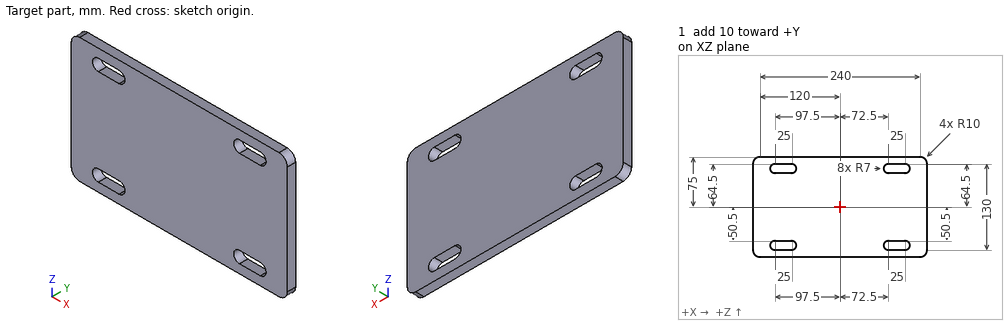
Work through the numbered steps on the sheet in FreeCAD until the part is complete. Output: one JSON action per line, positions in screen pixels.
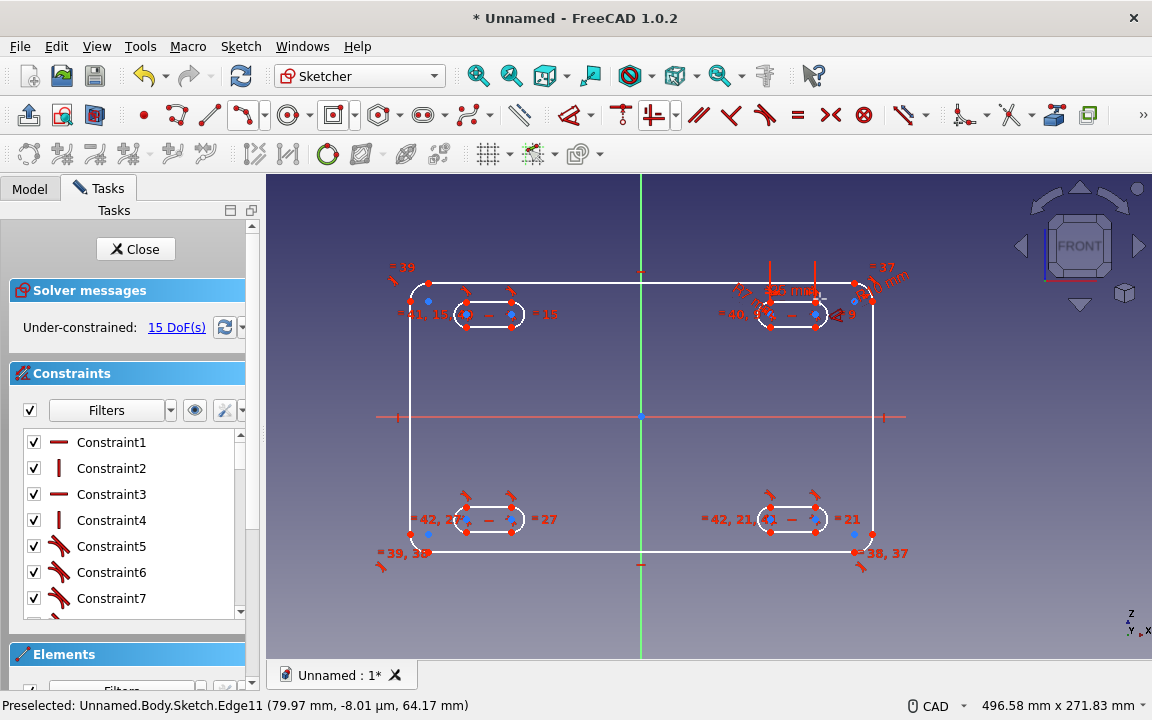
{"action": "left_click", "coordinate": [480, 302]}
{"action": "left_click", "coordinate": [489, 268]}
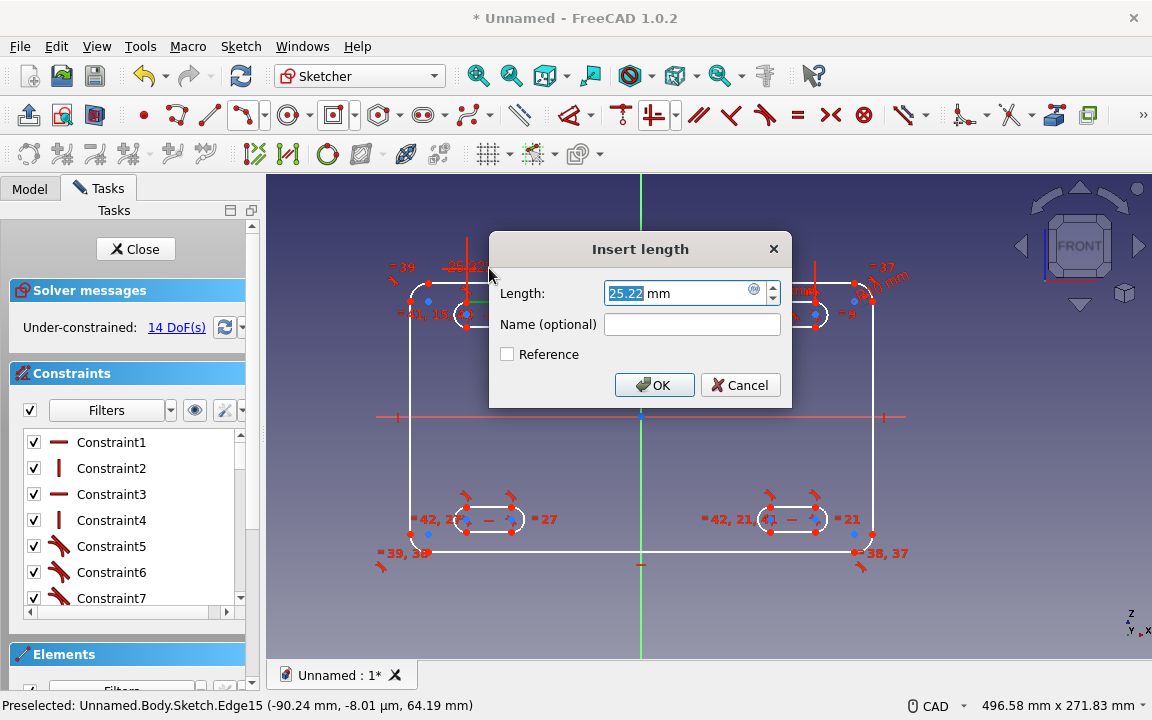
{"action": "type", "text": "25"}
{"action": "key", "text": "Return"}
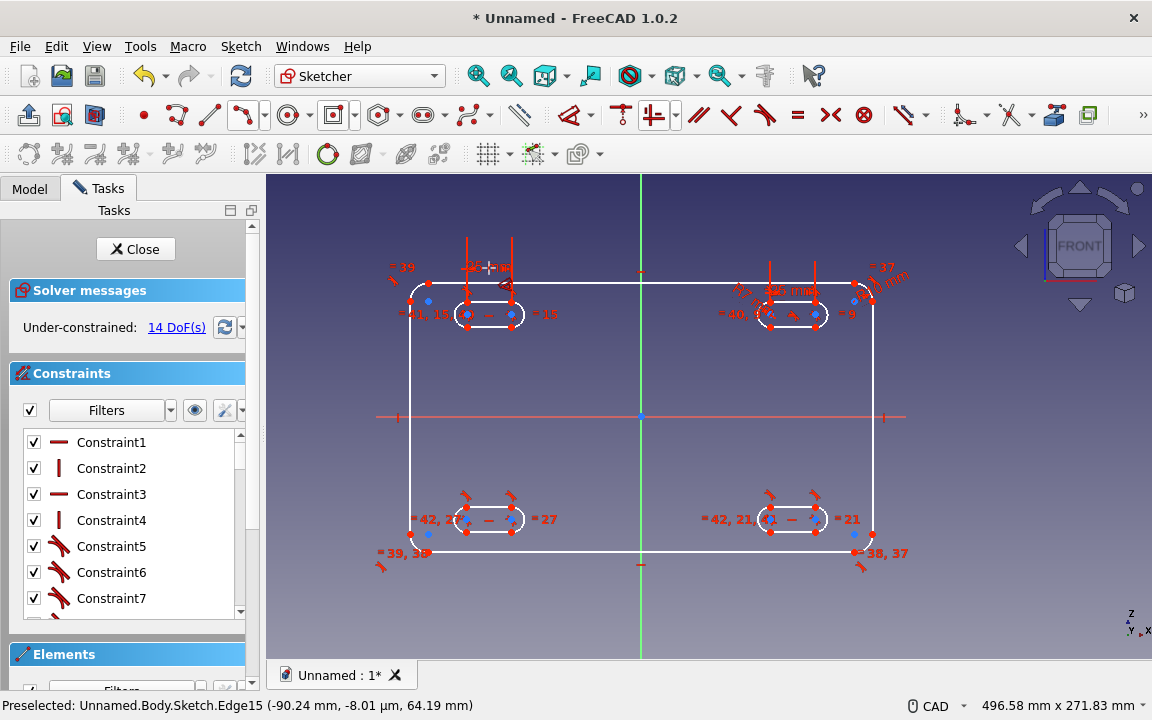
{"action": "left_click", "coordinate": [784, 507]}
{"action": "left_click", "coordinate": [793, 473]}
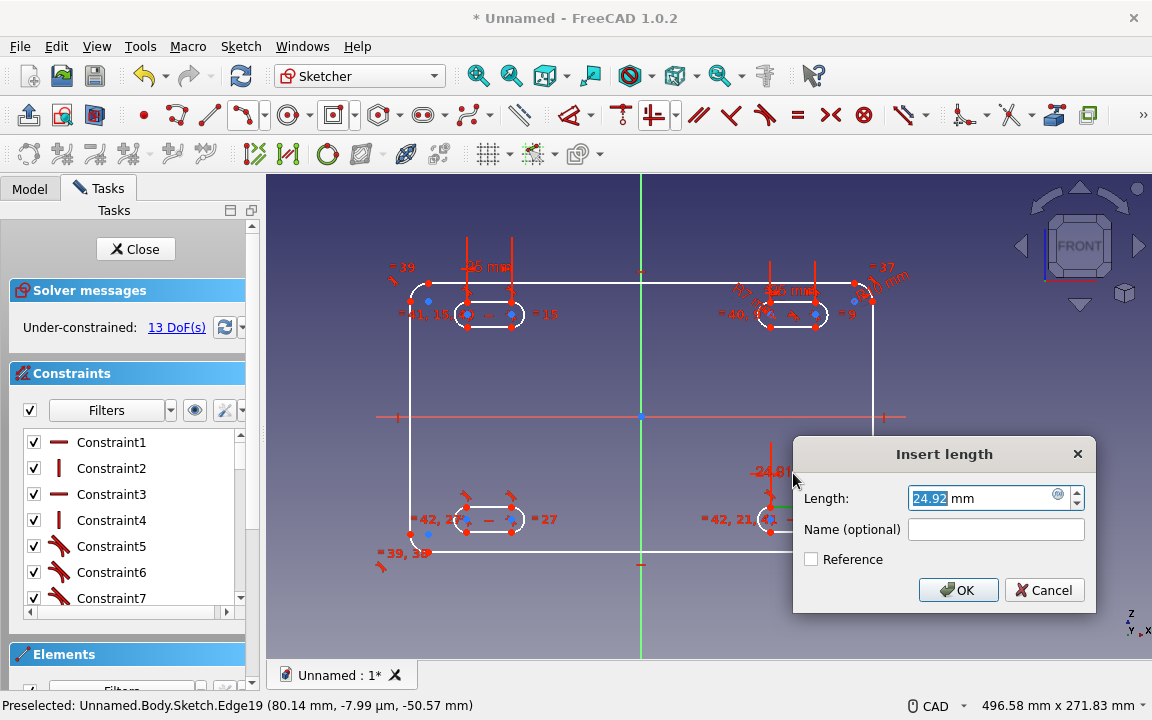
{"action": "type", "text": "25"}
{"action": "key", "text": "Return"}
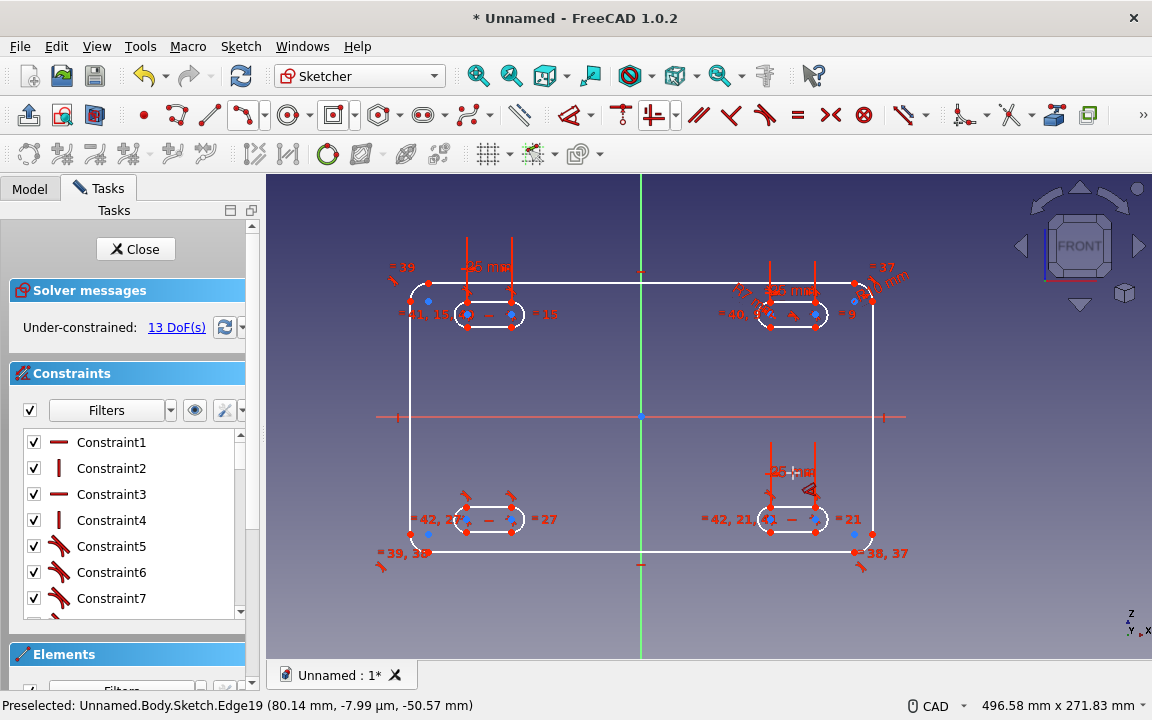
{"action": "left_click", "coordinate": [480, 507]}
{"action": "left_click", "coordinate": [489, 473]}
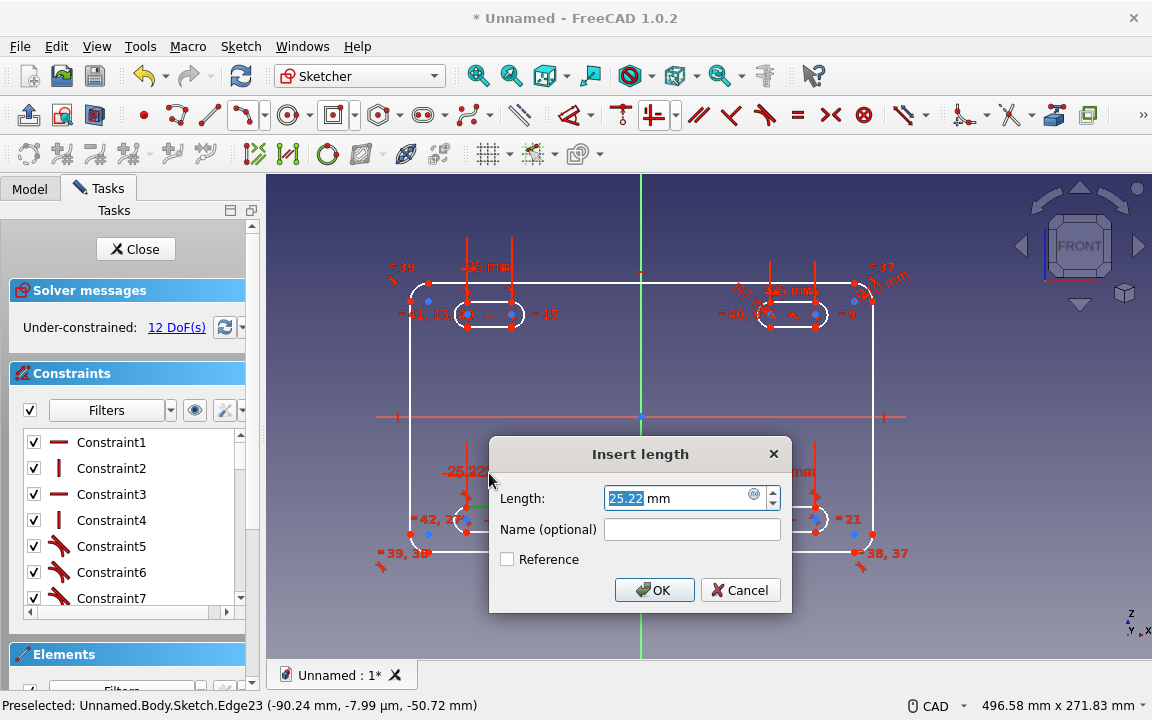
{"action": "type", "text": "25"}
{"action": "key", "text": "Return"}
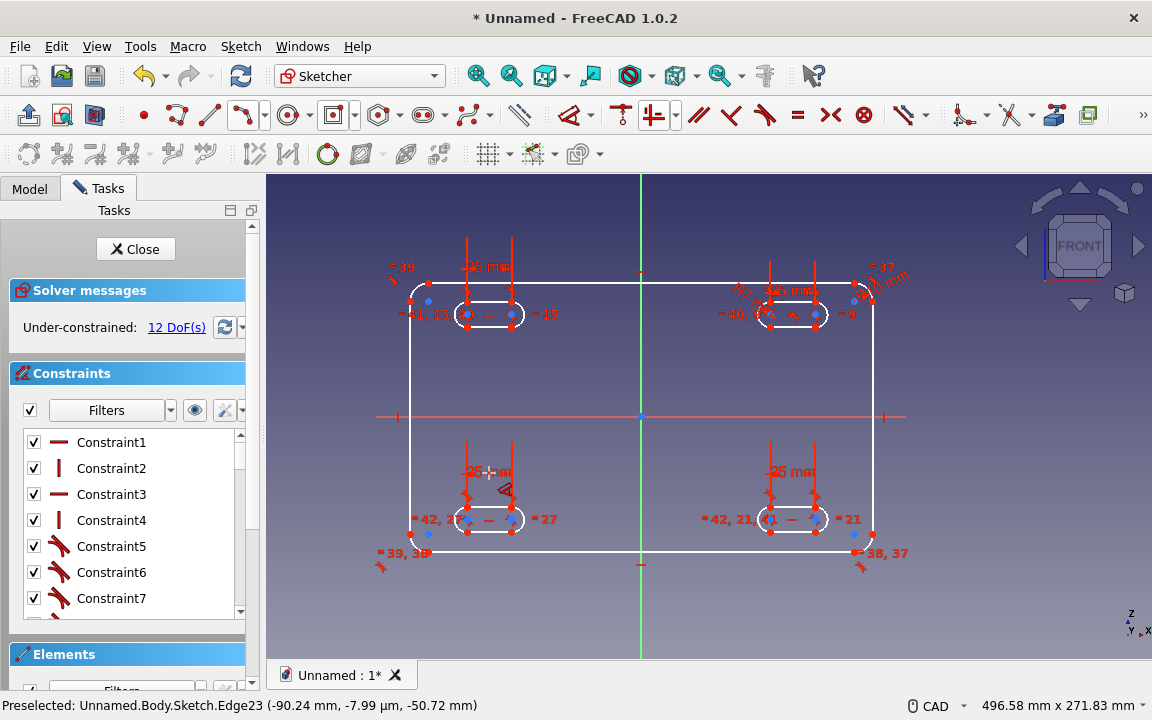
{"action": "left_click", "coordinate": [556, 283]}
{"action": "left_click", "coordinate": [740, 249]}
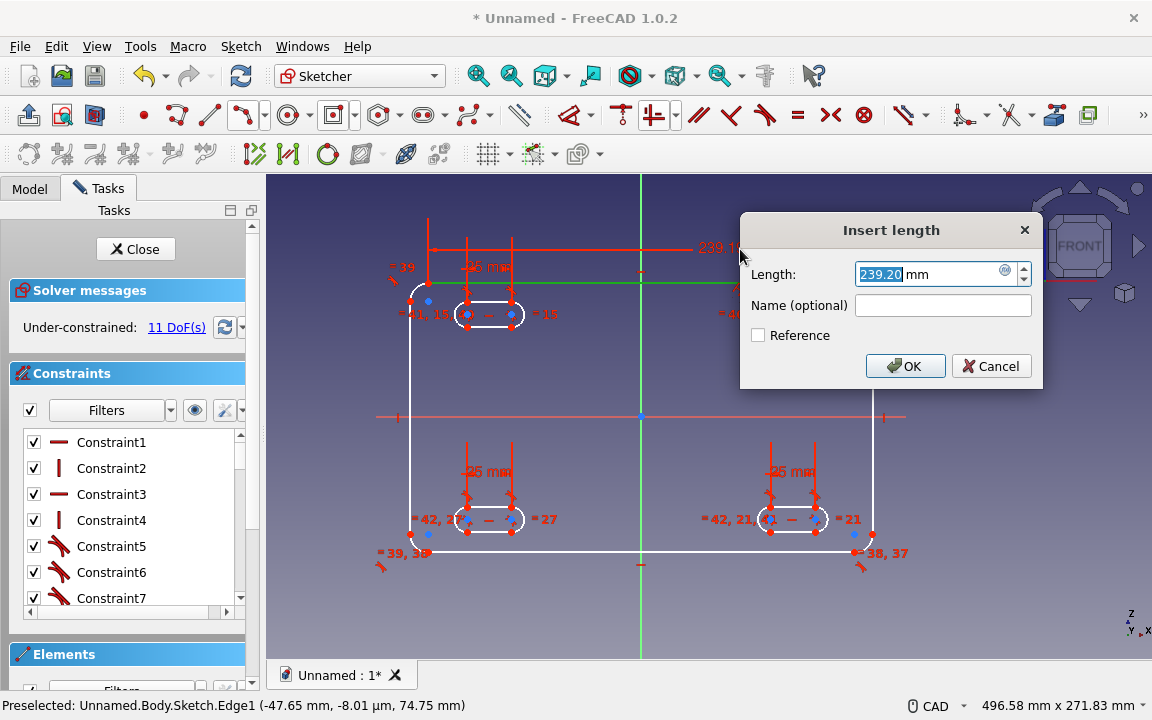
{"action": "type", "text": "240"}
{"action": "key", "text": "Return"}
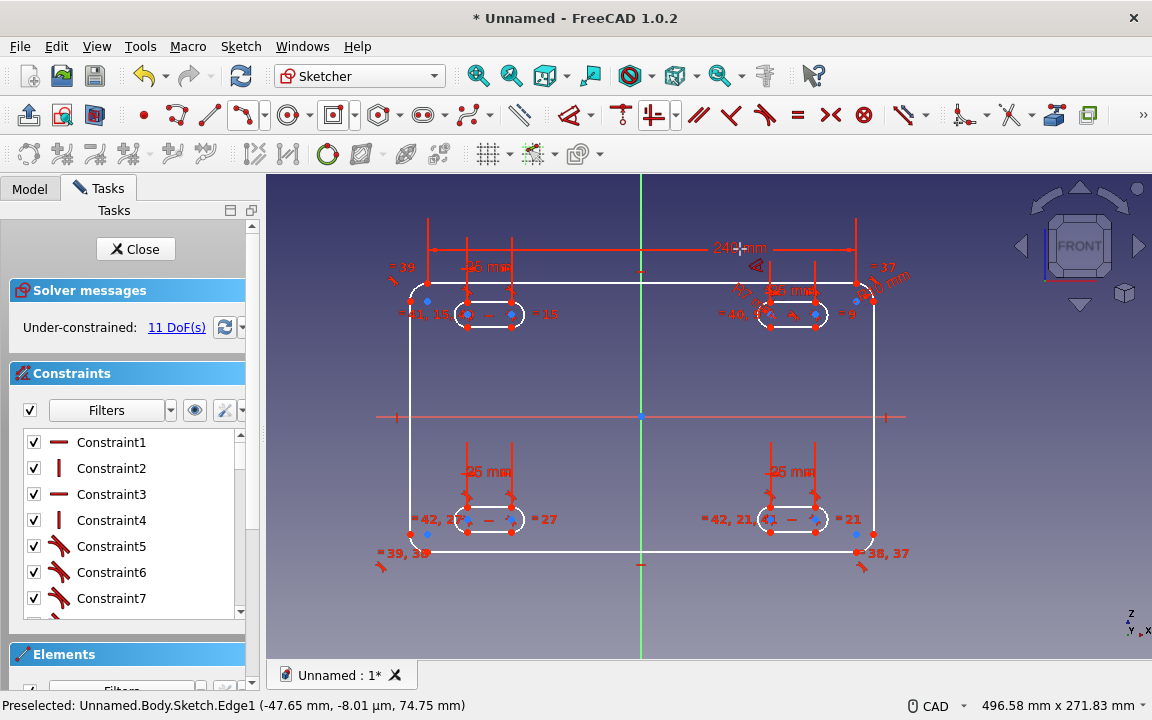
{"action": "left_click", "coordinate": [874, 371]}
{"action": "left_click", "coordinate": [908, 364]}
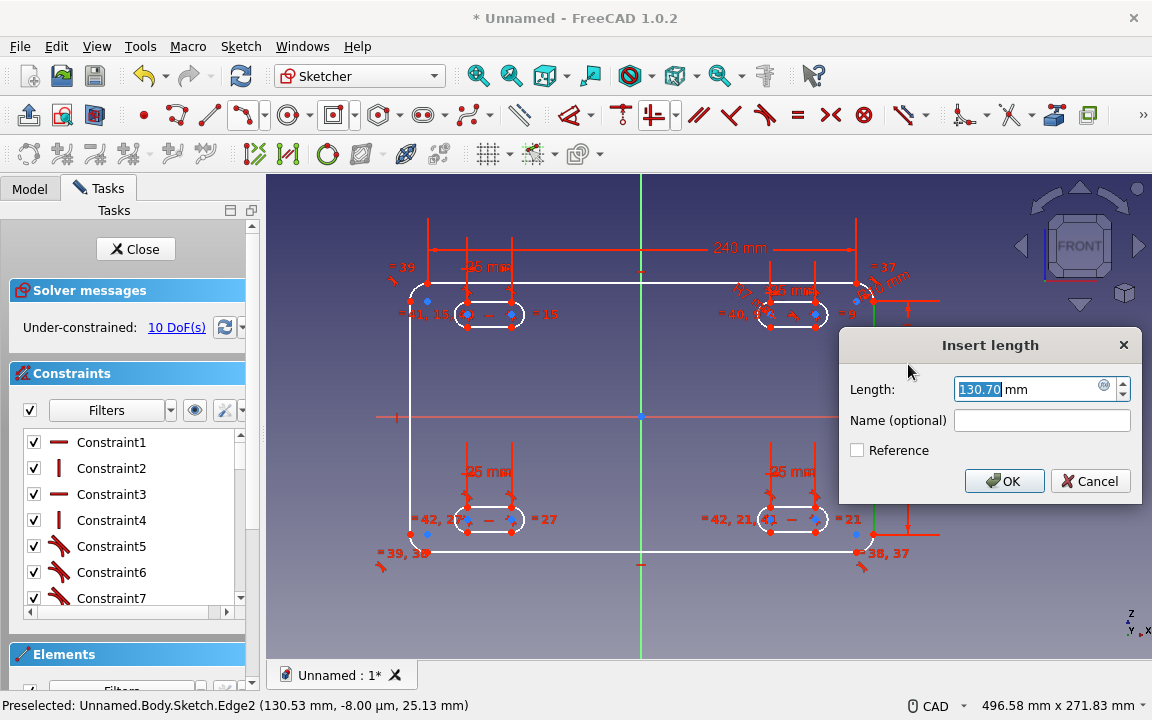
{"action": "type", "text": "130"}
{"action": "key", "text": "Return"}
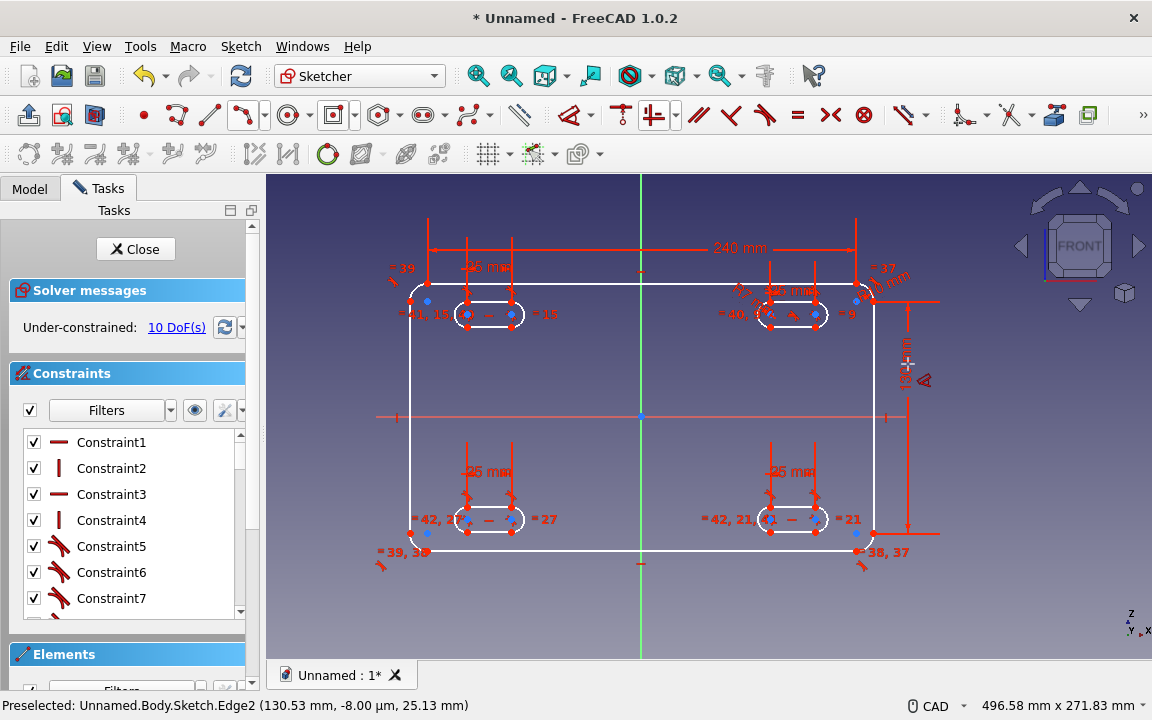
{"action": "left_click", "coordinate": [428, 284]}
{"action": "left_click", "coordinate": [394, 350]}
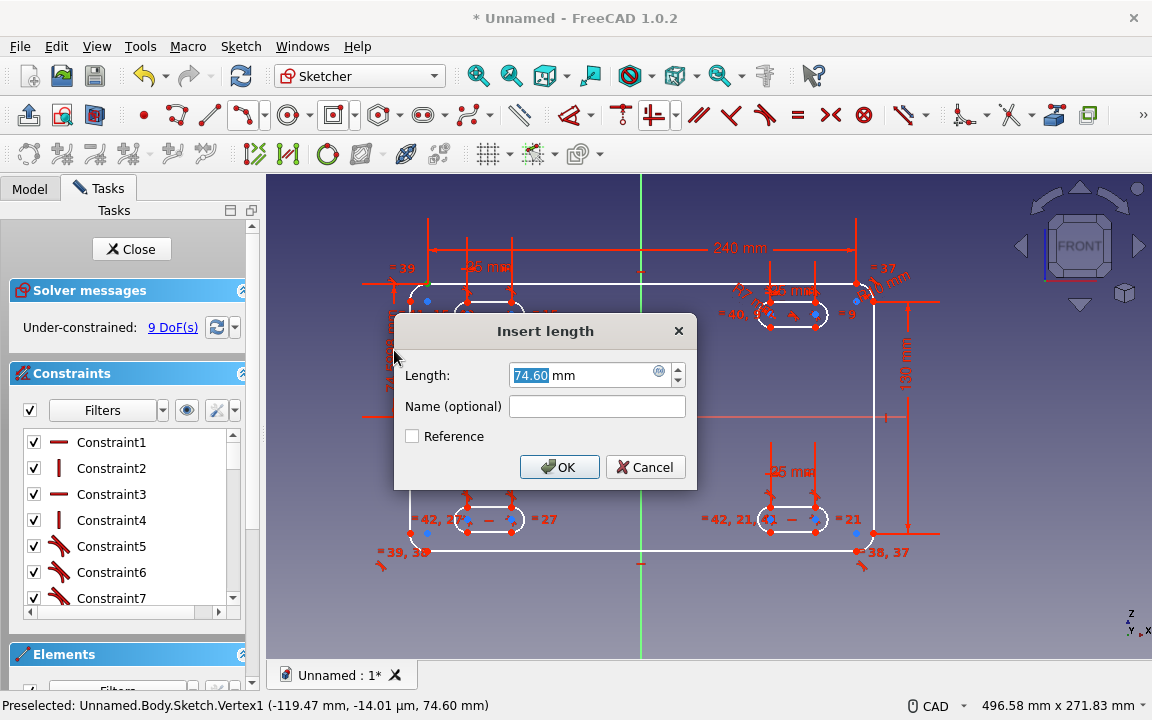
{"action": "type", "text": "75"}
{"action": "key", "text": "Return"}